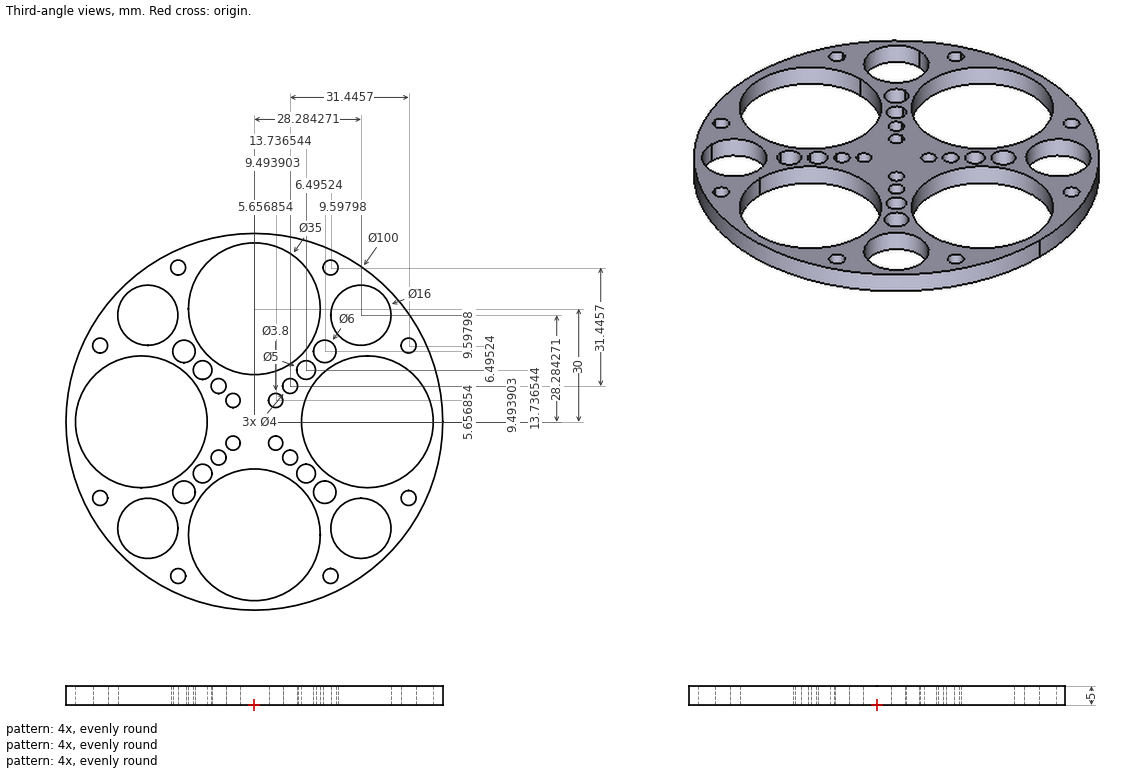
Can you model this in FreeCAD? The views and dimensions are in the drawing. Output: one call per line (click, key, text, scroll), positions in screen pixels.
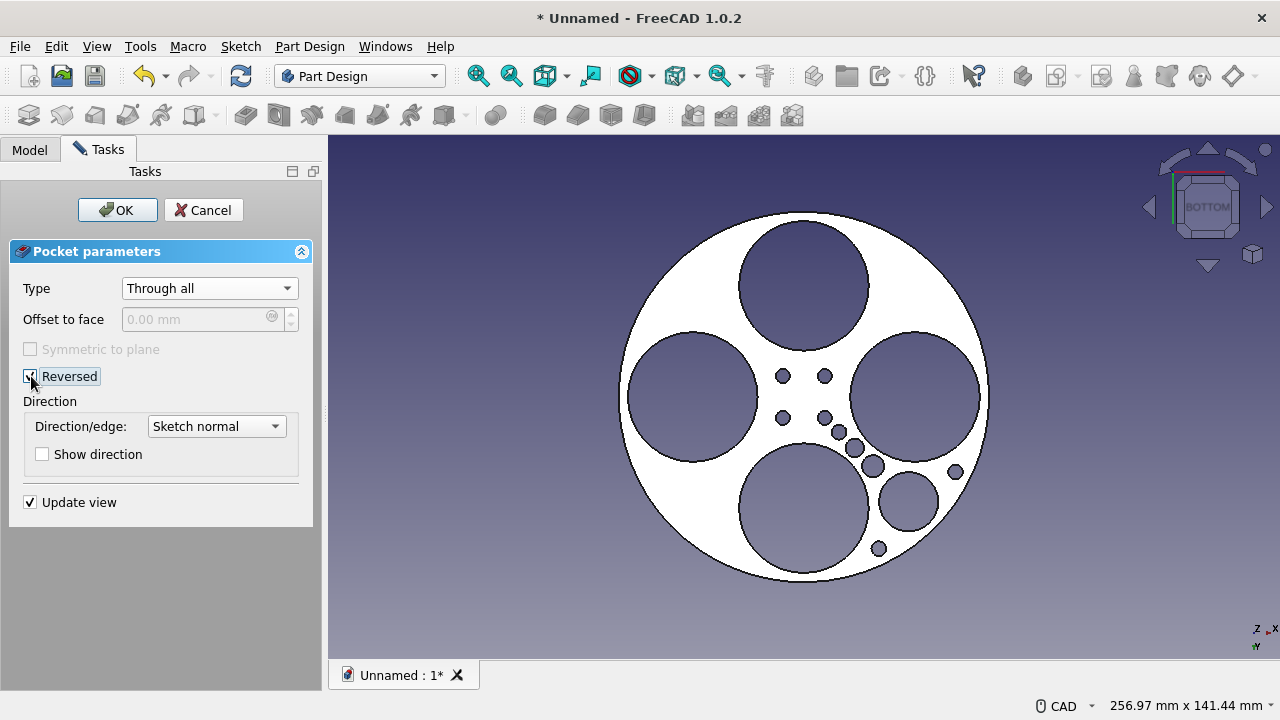
click(118, 210)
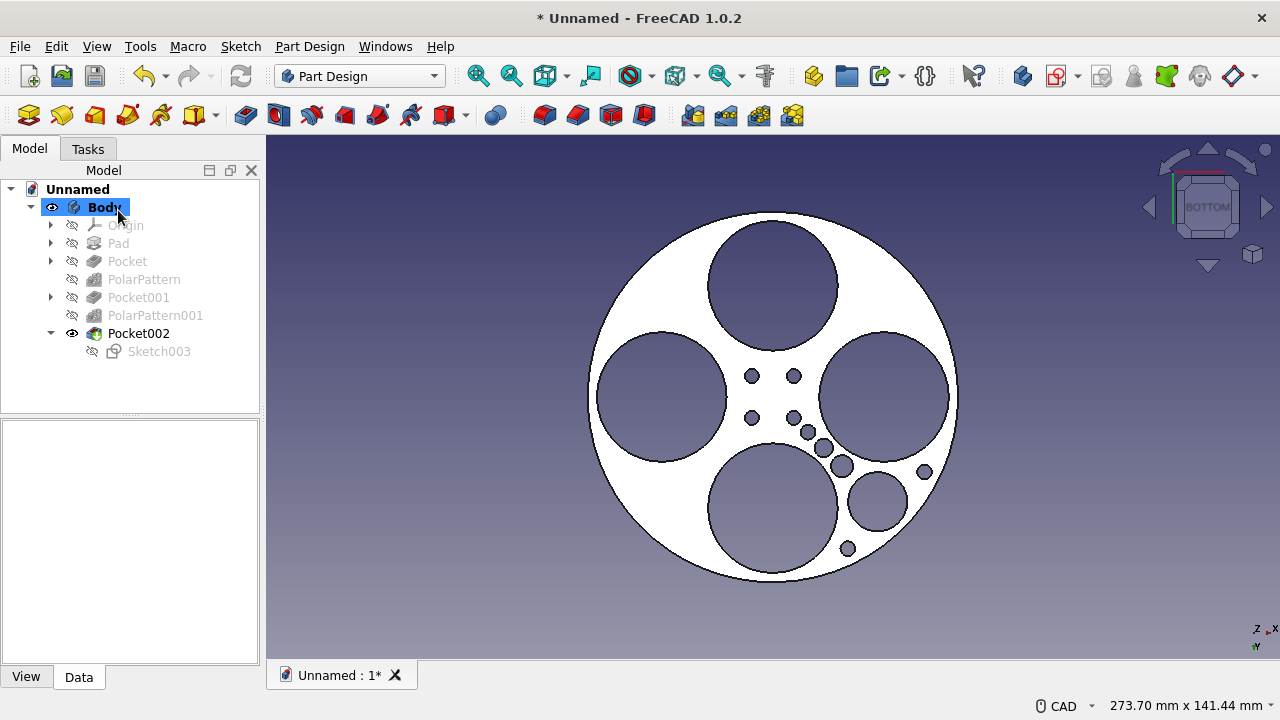
click(117, 333)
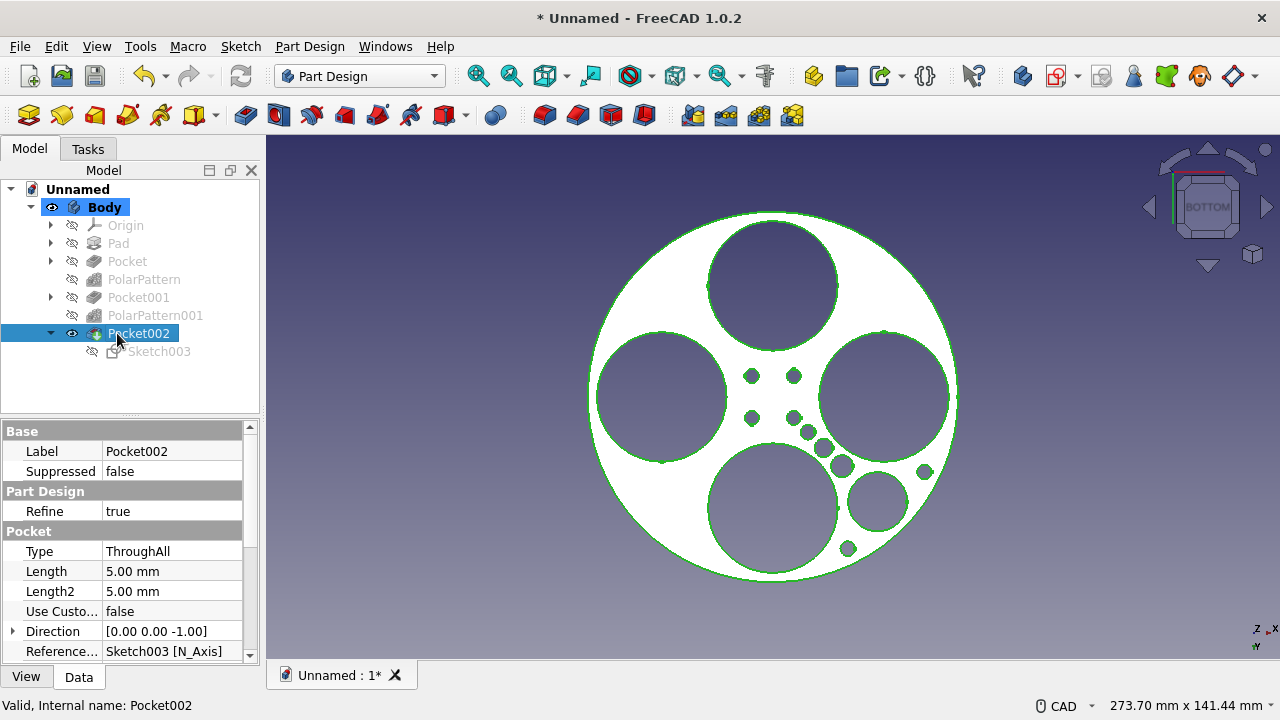
click(759, 116)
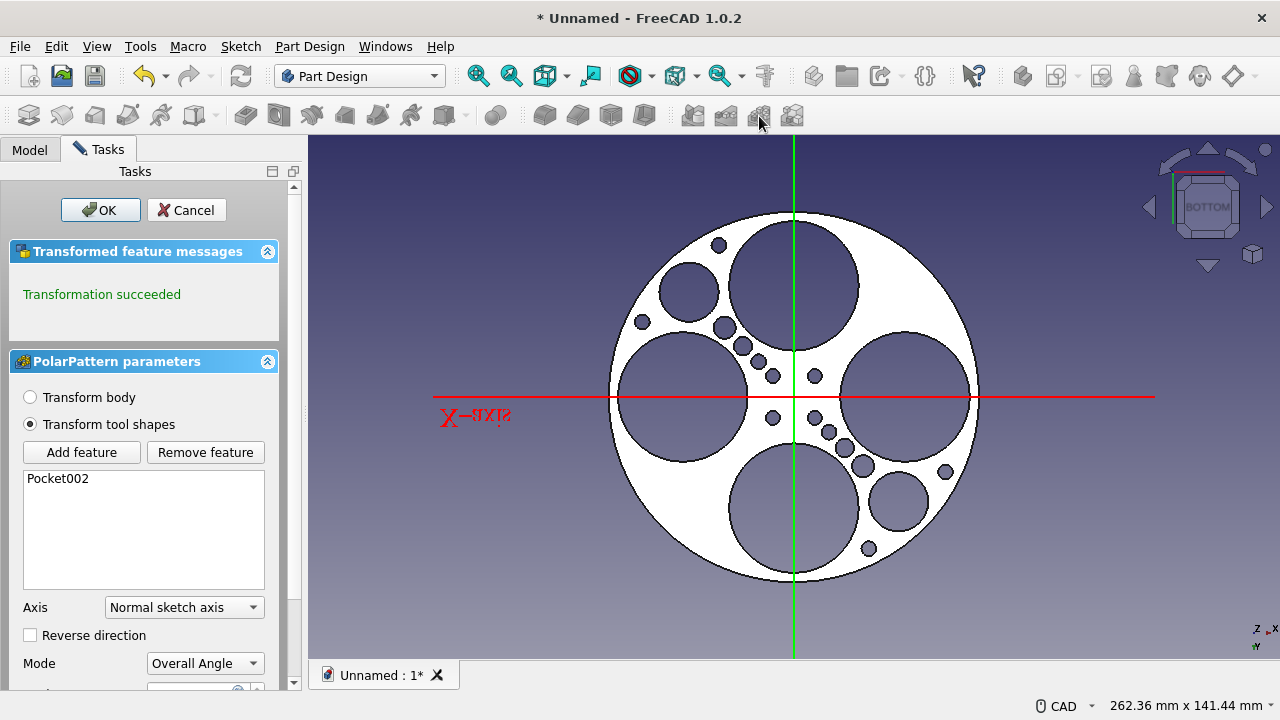
click(185, 608)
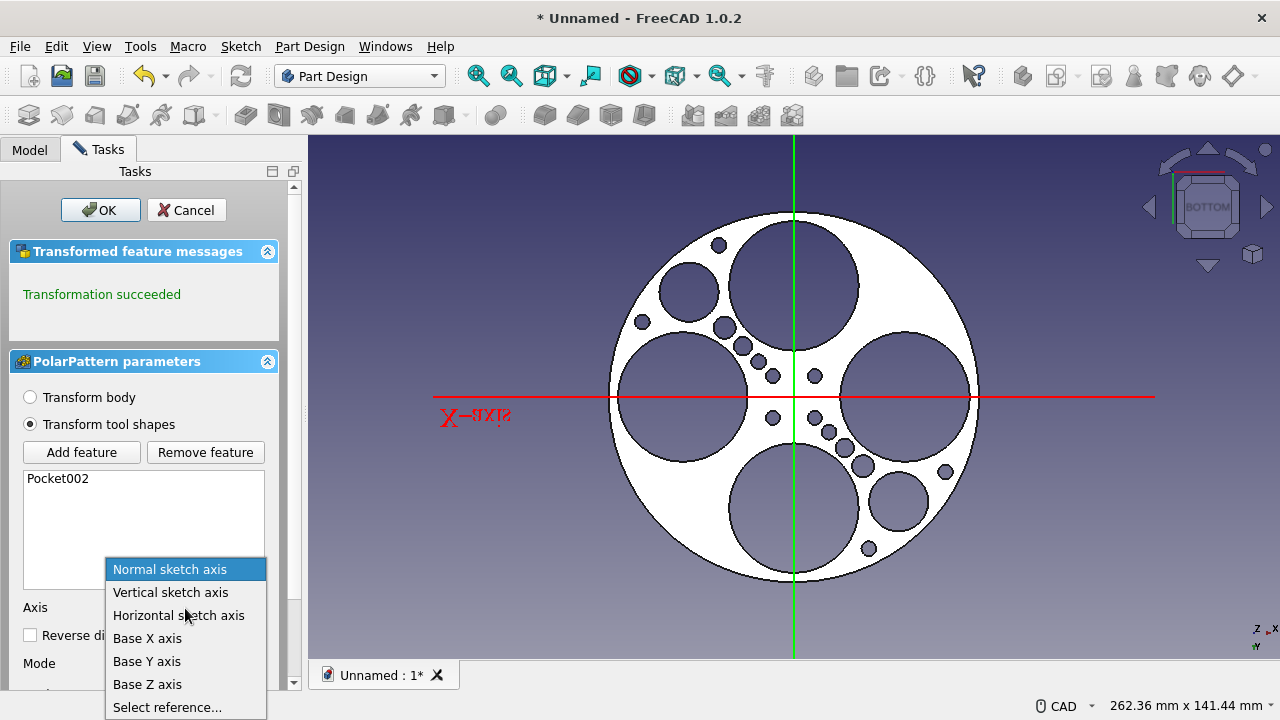
click(184, 684)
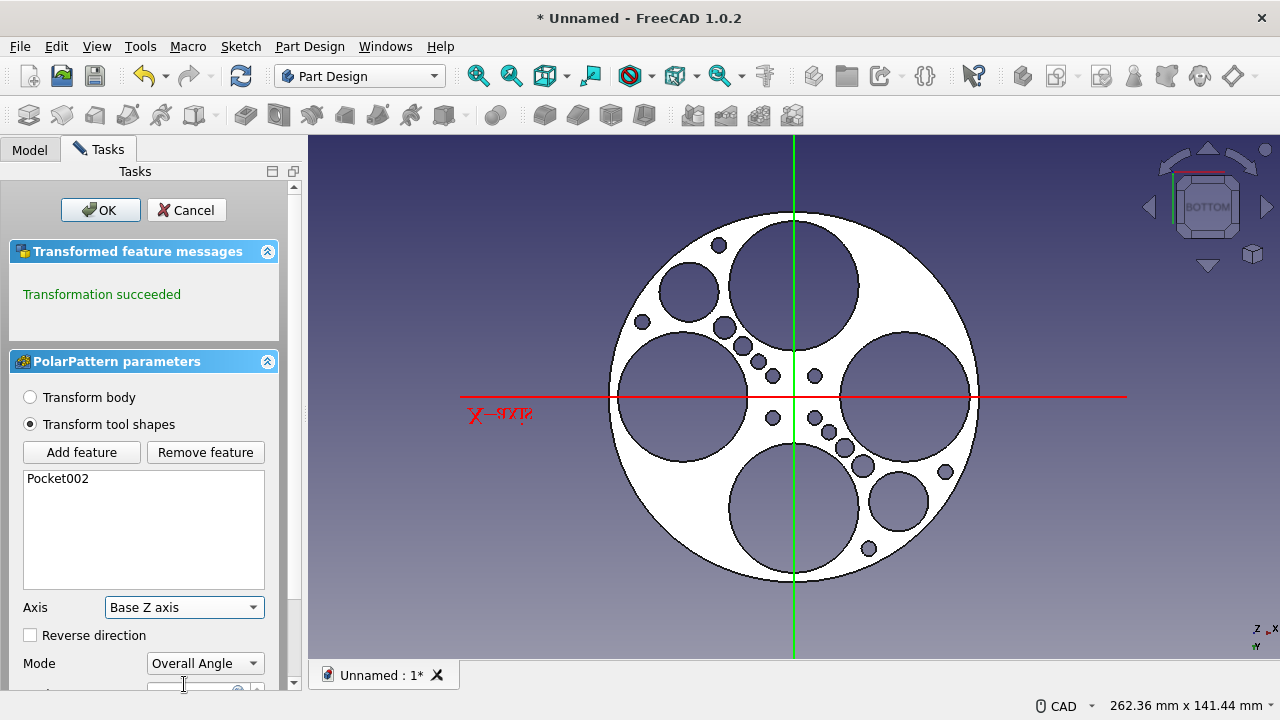
scroll(294, 436, down, 2)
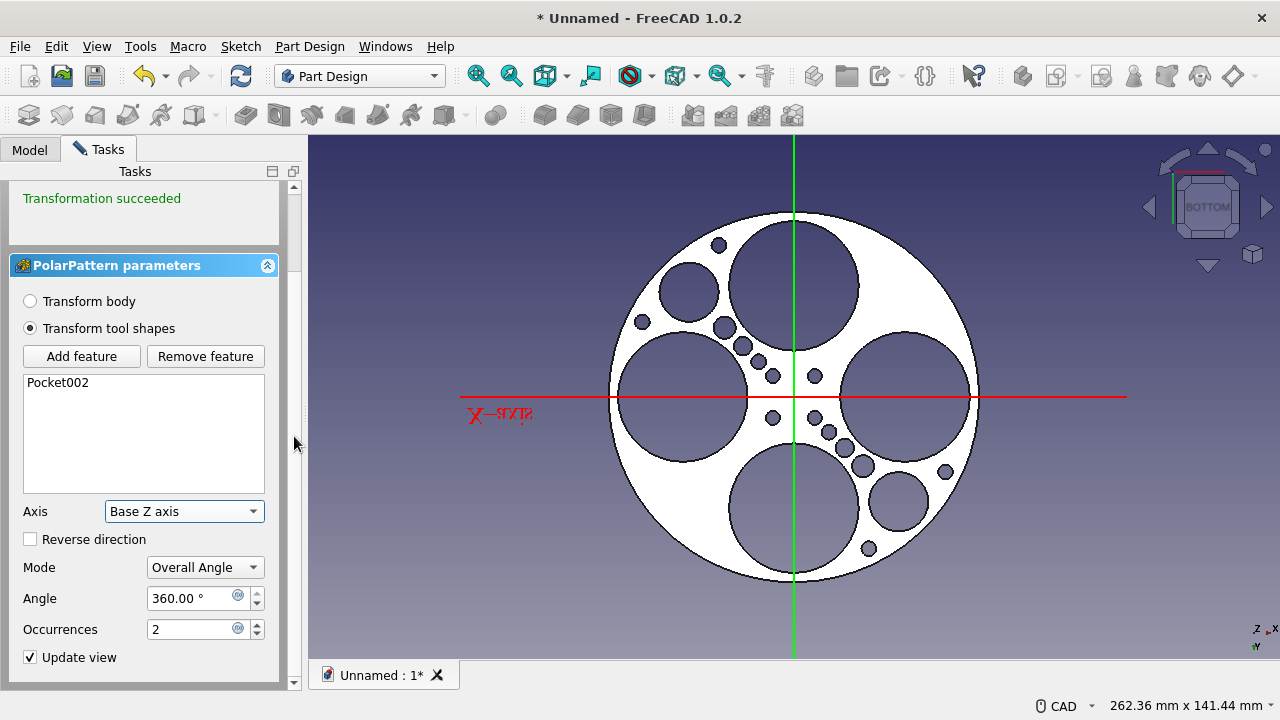
triple_click(199, 630)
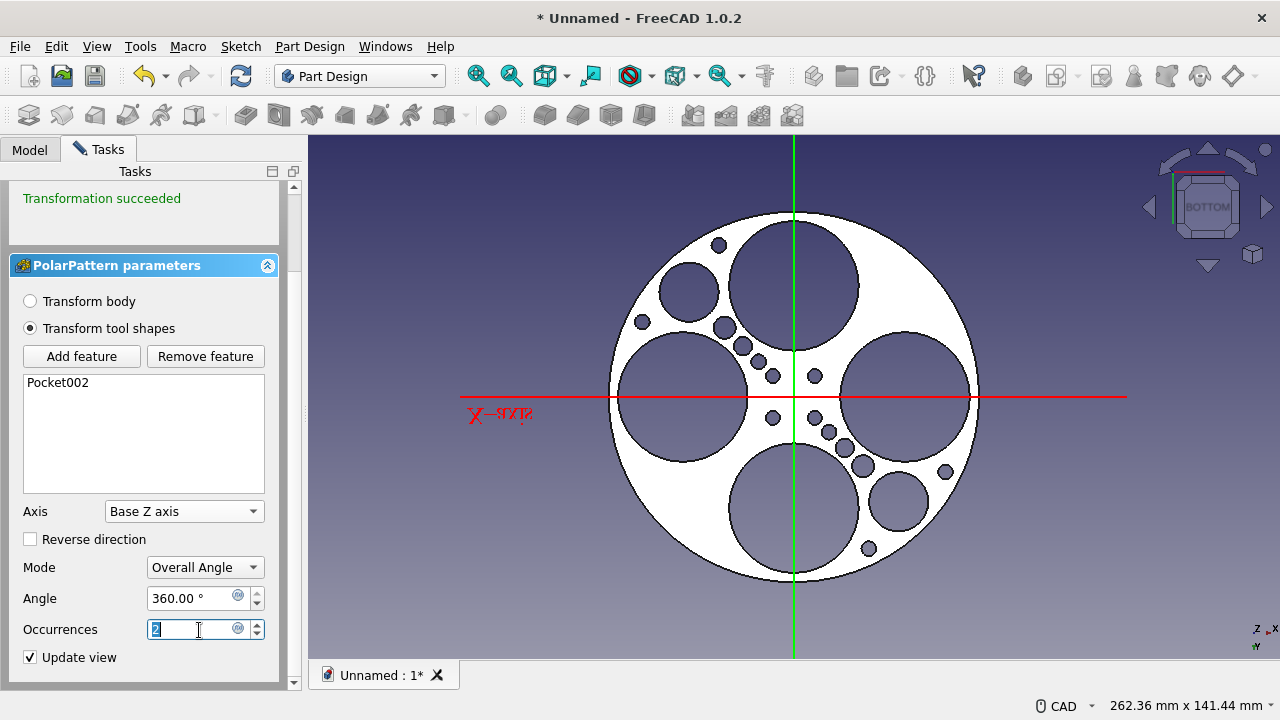
text(4)
key(Tab)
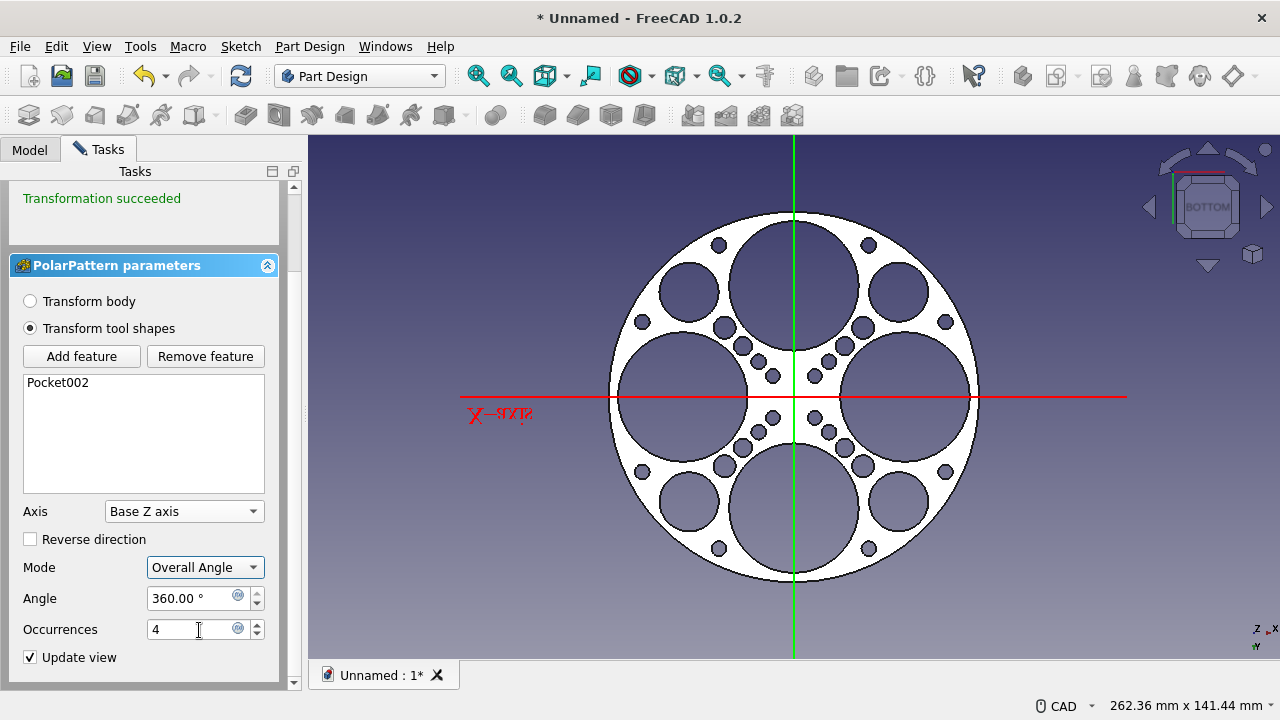
scroll(294, 436, up, 3)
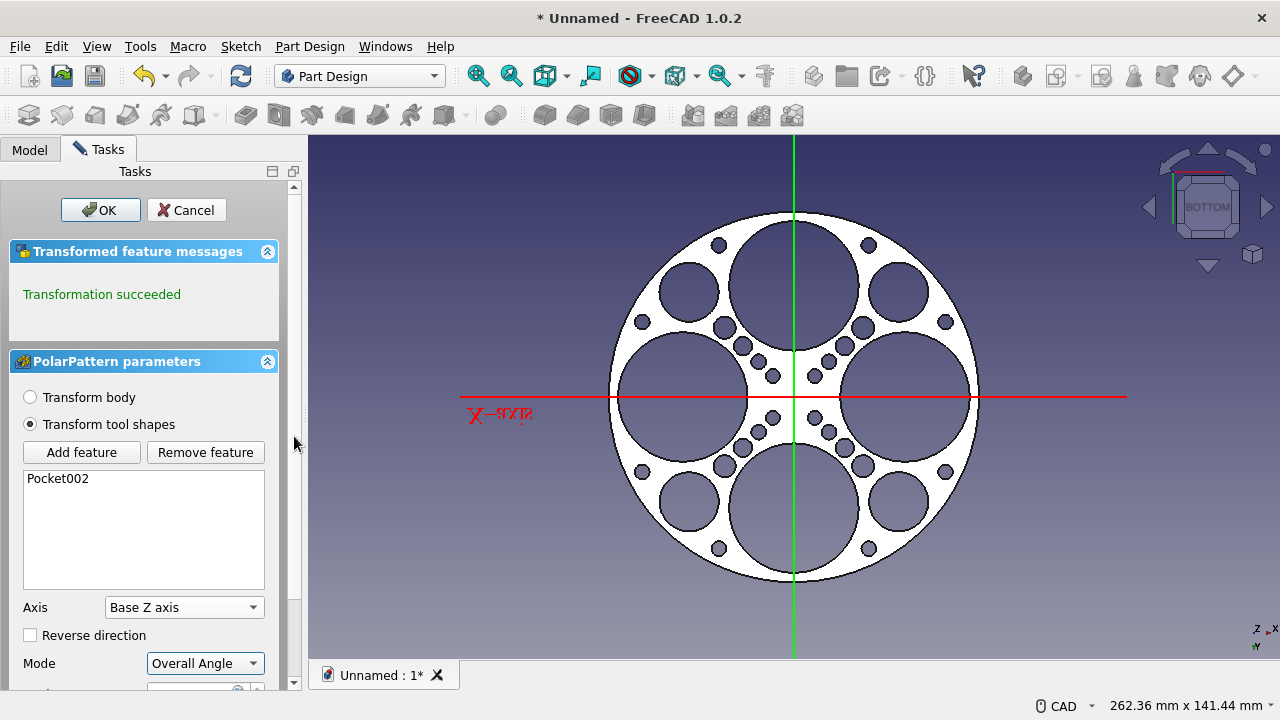
click(101, 210)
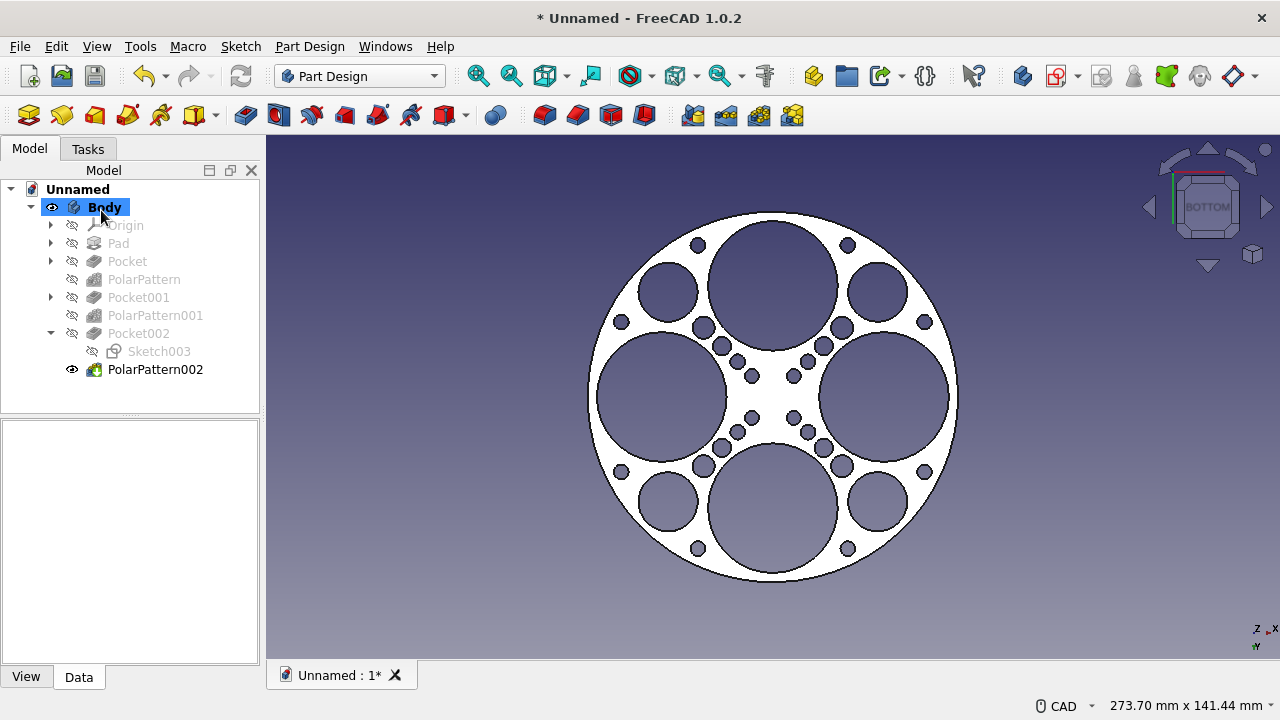
key(0)